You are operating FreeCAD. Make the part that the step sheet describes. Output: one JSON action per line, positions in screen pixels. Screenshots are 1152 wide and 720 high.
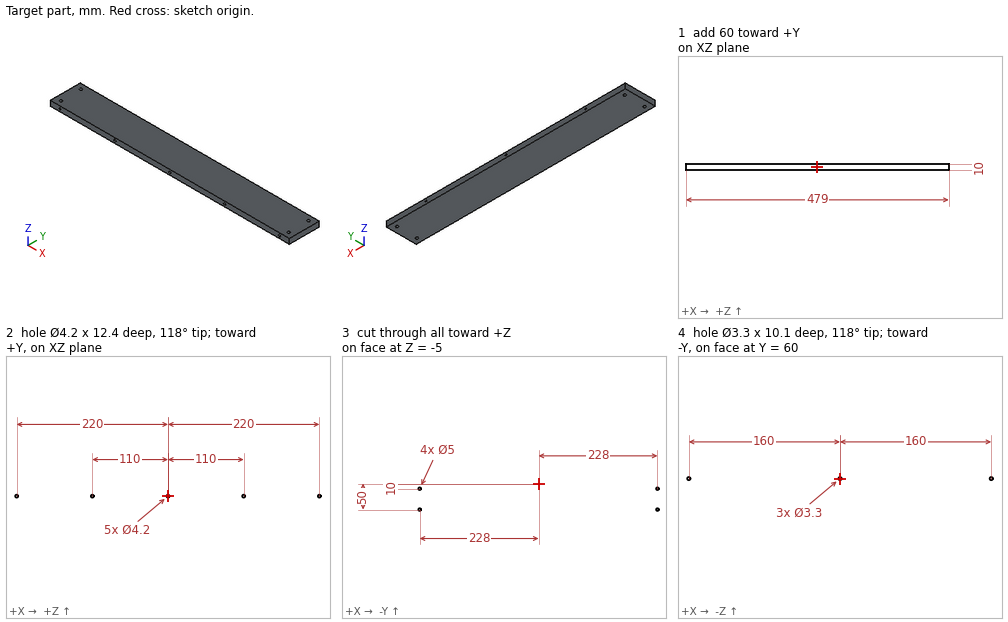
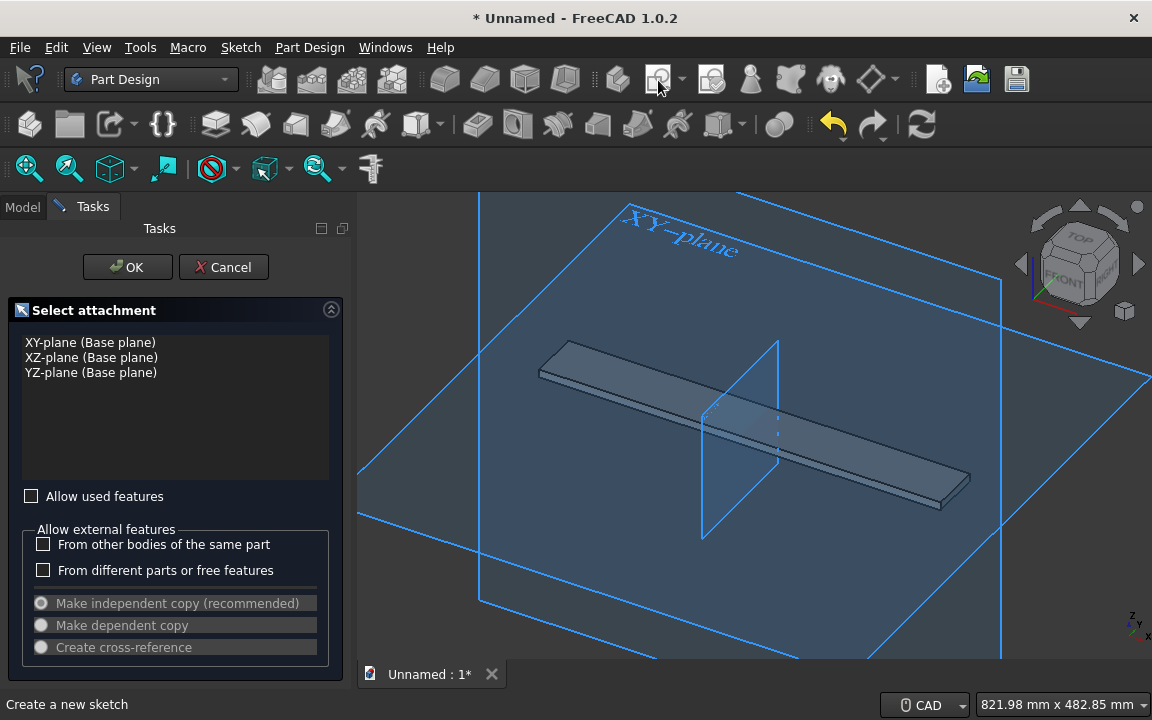
{"action": "left_click", "coordinate": [82, 358]}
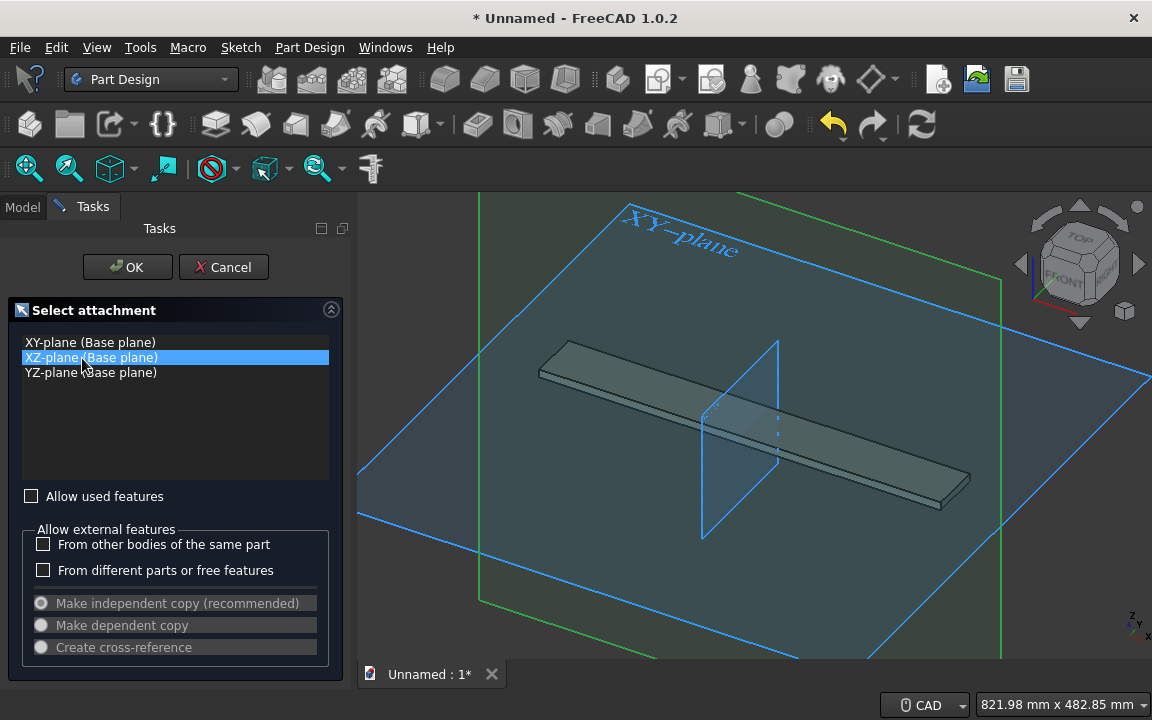
{"action": "left_click", "coordinate": [128, 267]}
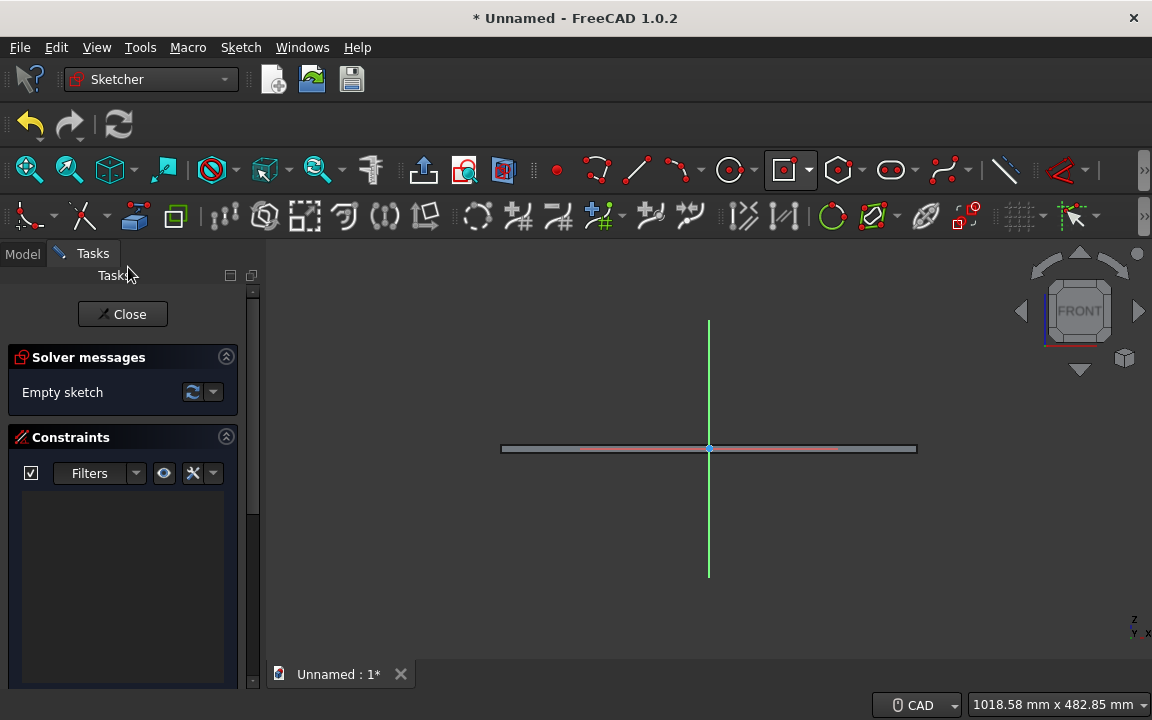
{"action": "left_click", "coordinate": [730, 170]}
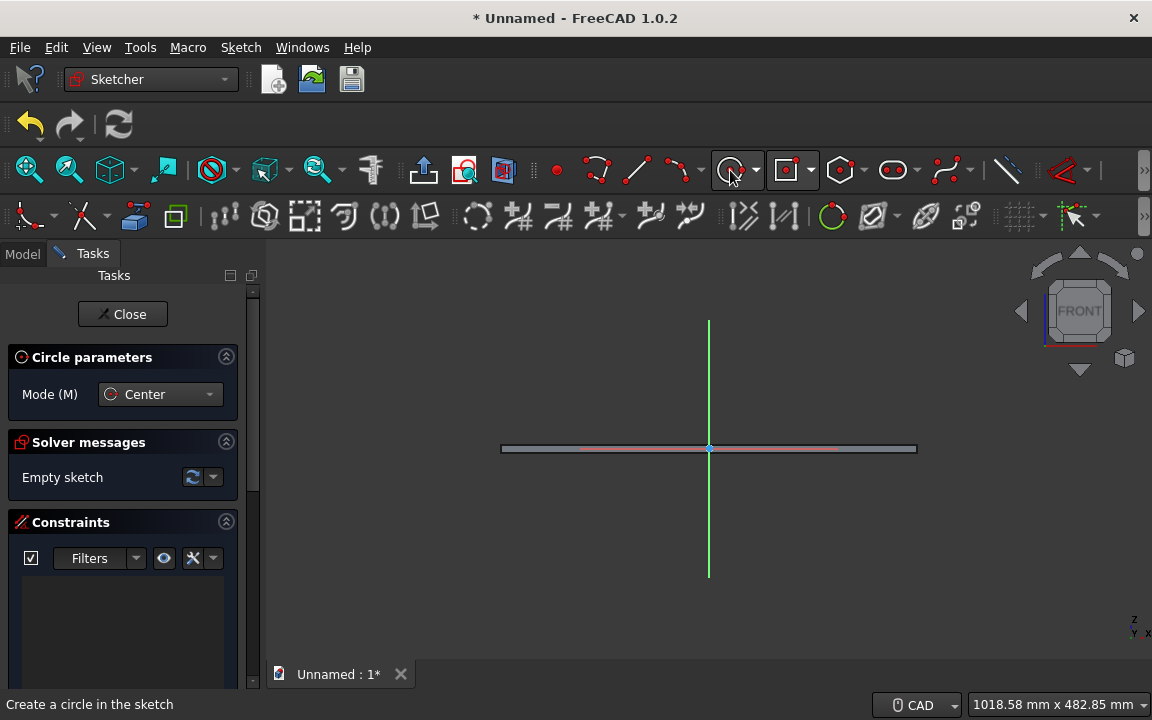
{"action": "scroll", "coordinate": [709, 449], "scroll_direction": "up", "scroll_amount": 13}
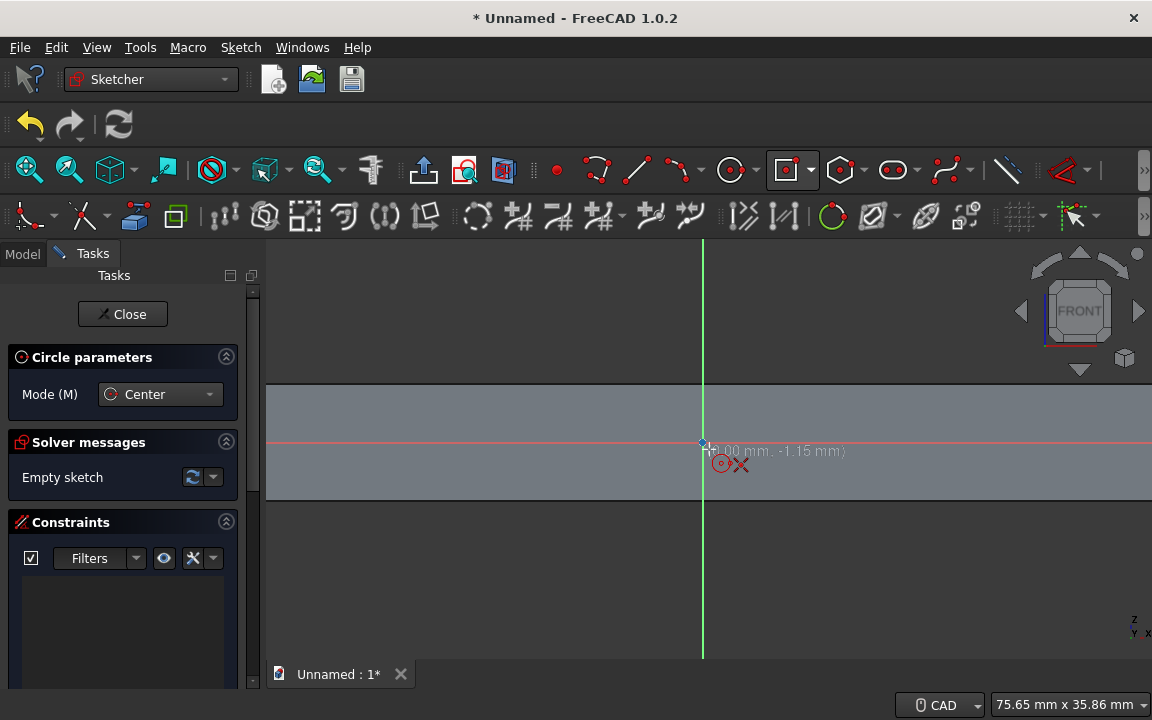
{"action": "scroll", "coordinate": [634, 450], "scroll_direction": "down", "scroll_amount": 12}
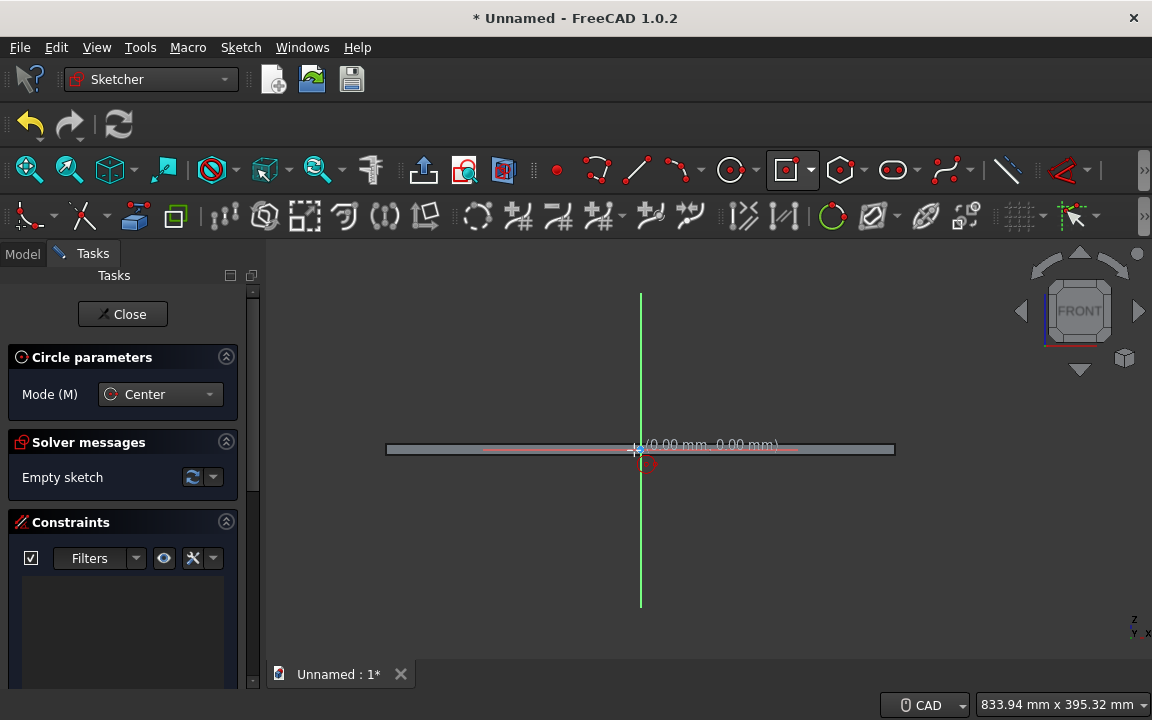
{"action": "left_click", "coordinate": [641, 450]}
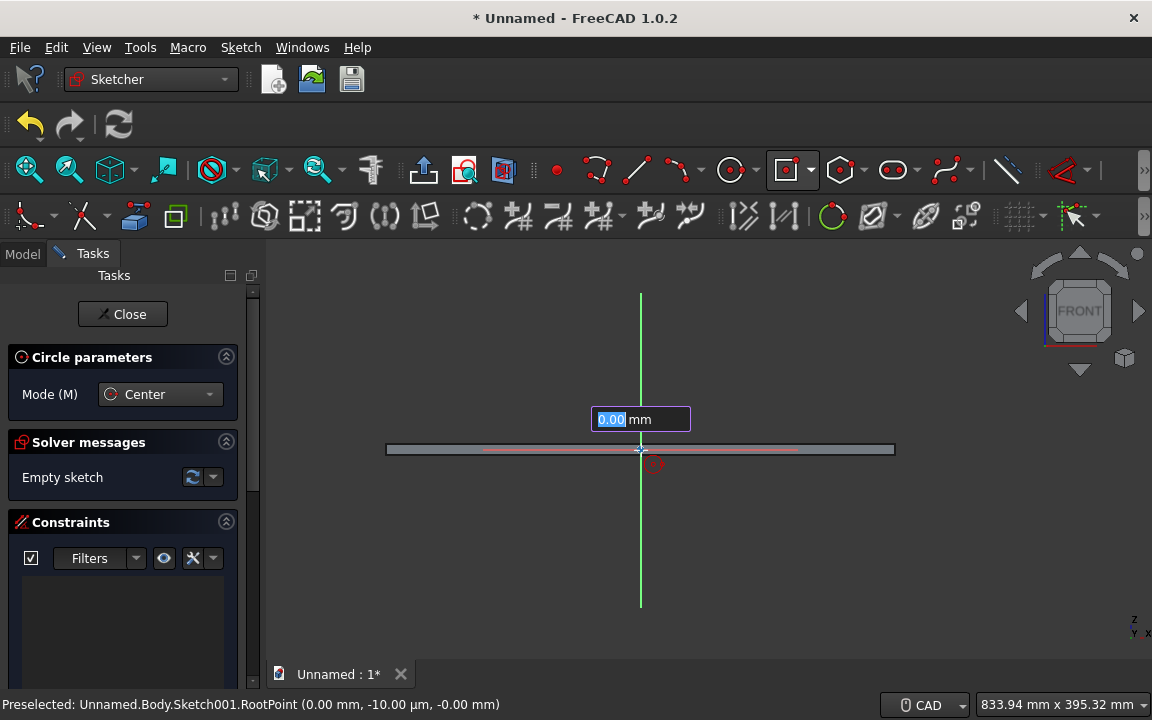
{"action": "scroll", "coordinate": [642, 448], "scroll_direction": "up", "scroll_amount": 12}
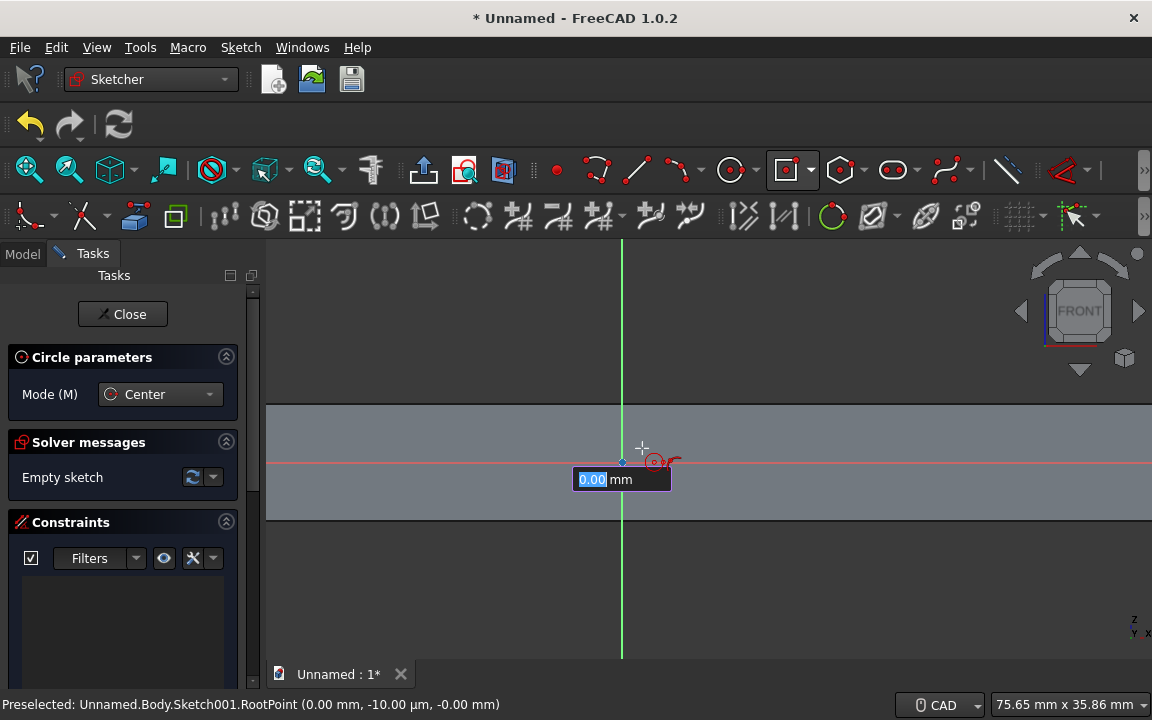
{"action": "left_click", "coordinate": [640, 445]}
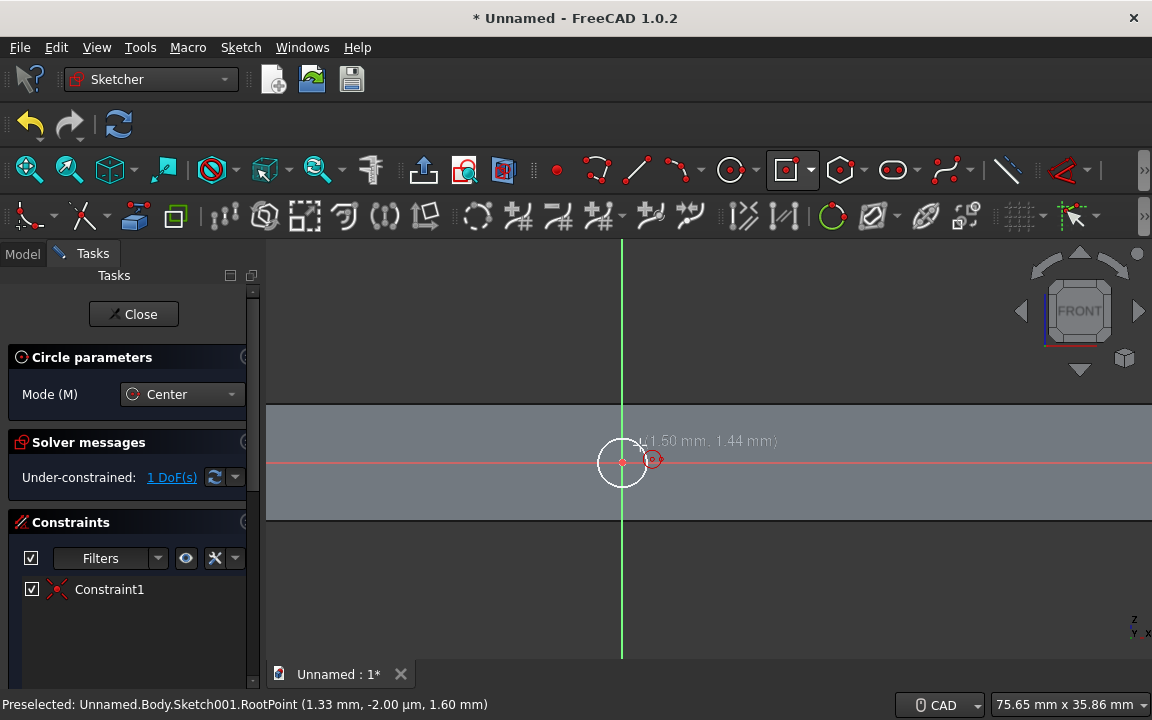
{"action": "scroll", "coordinate": [642, 448], "scroll_direction": "down", "scroll_amount": 12}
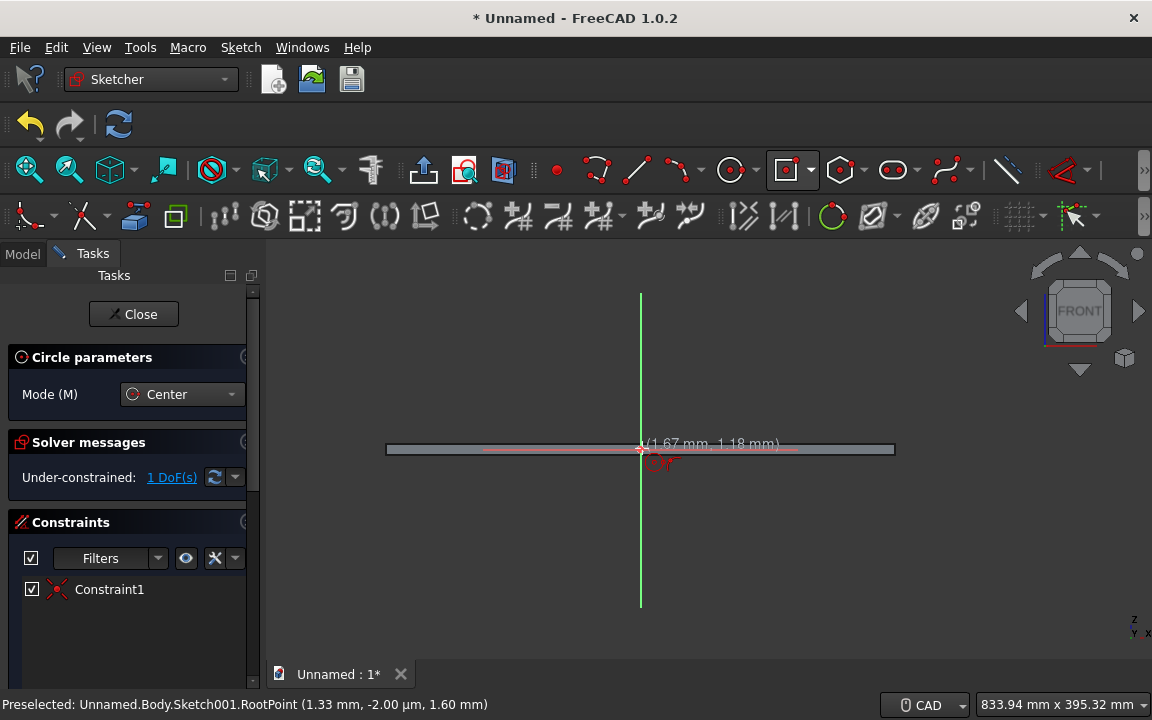
{"action": "scroll", "coordinate": [757, 450], "scroll_direction": "up", "scroll_amount": 12}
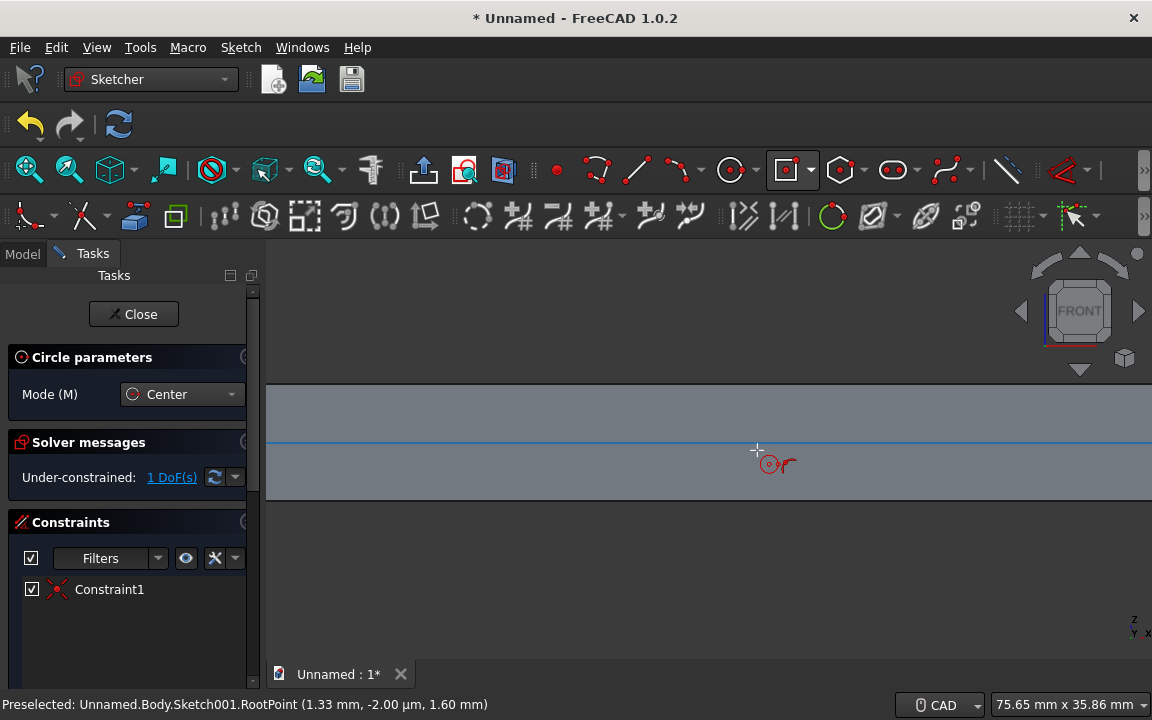
{"action": "scroll", "coordinate": [757, 450], "scroll_direction": "down", "scroll_amount": 12}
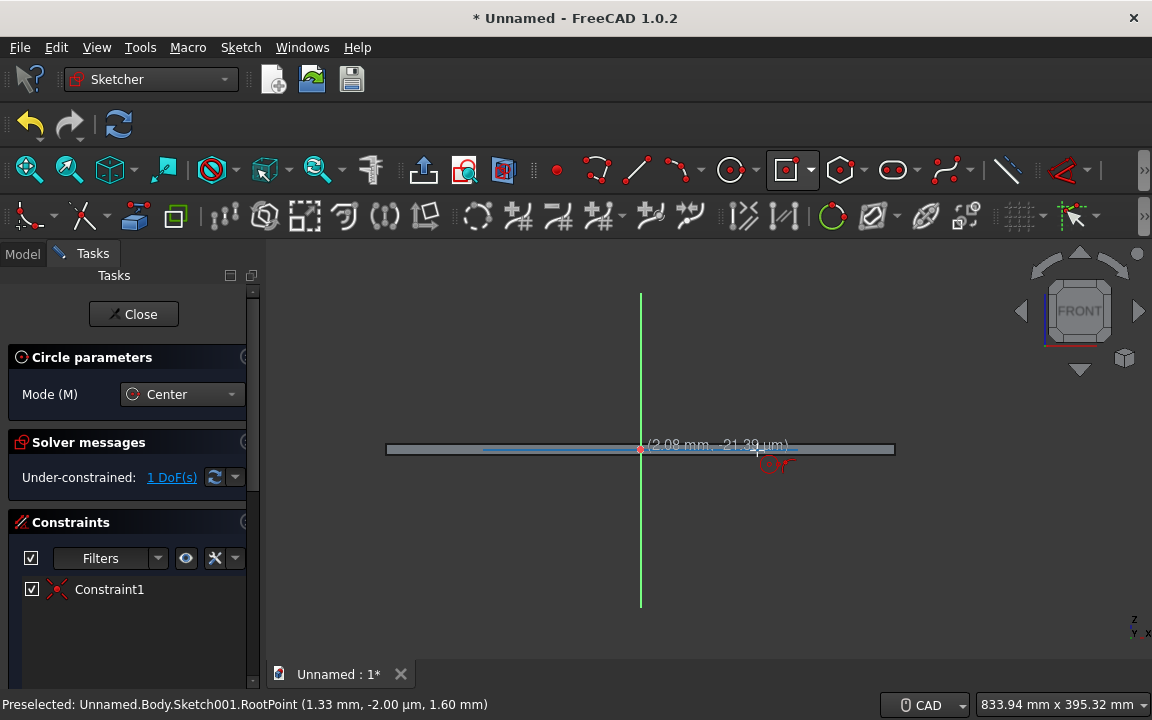
{"action": "left_click", "coordinate": [757, 450]}